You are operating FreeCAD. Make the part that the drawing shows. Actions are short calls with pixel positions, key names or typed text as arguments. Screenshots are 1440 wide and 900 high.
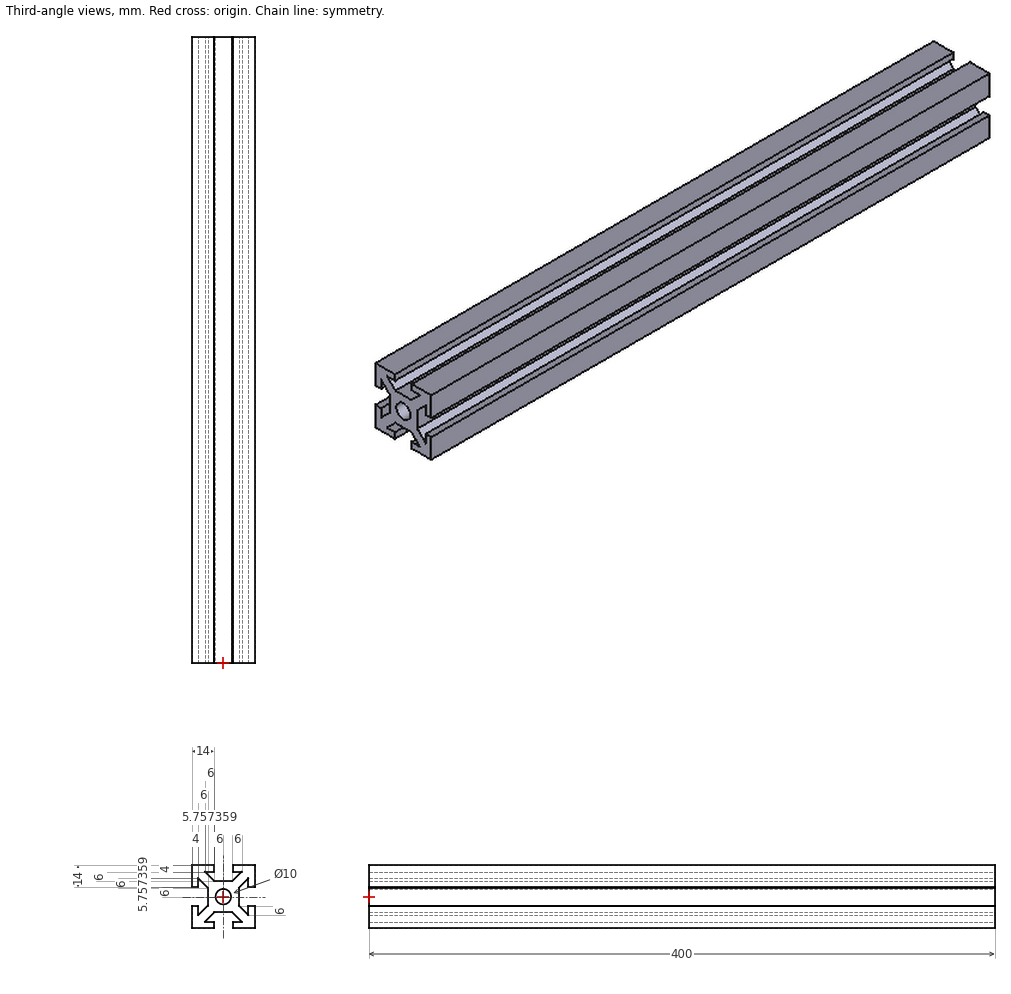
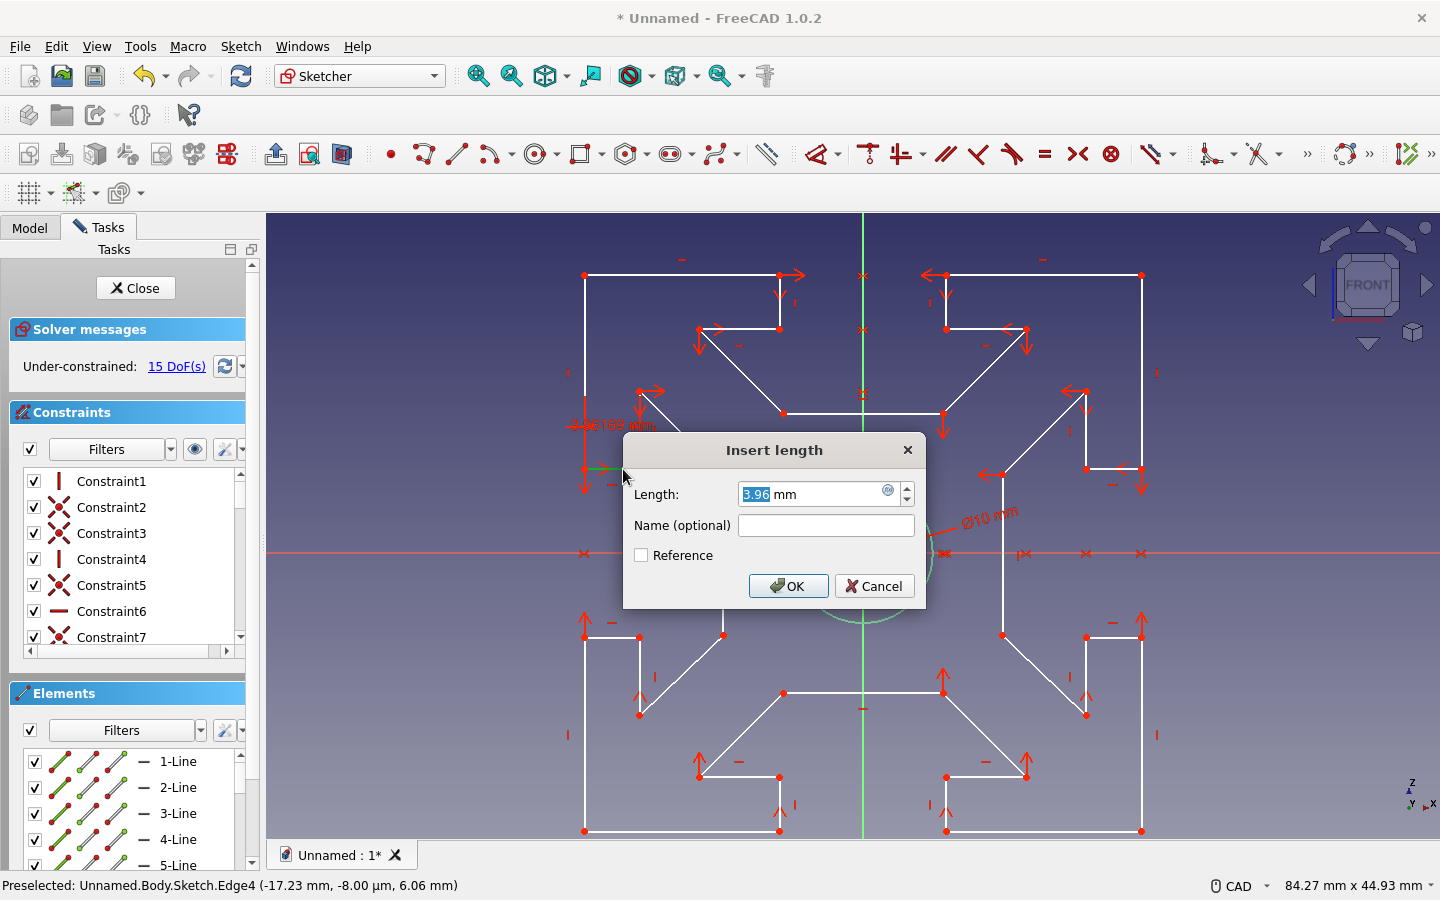
text(4)
key(Return)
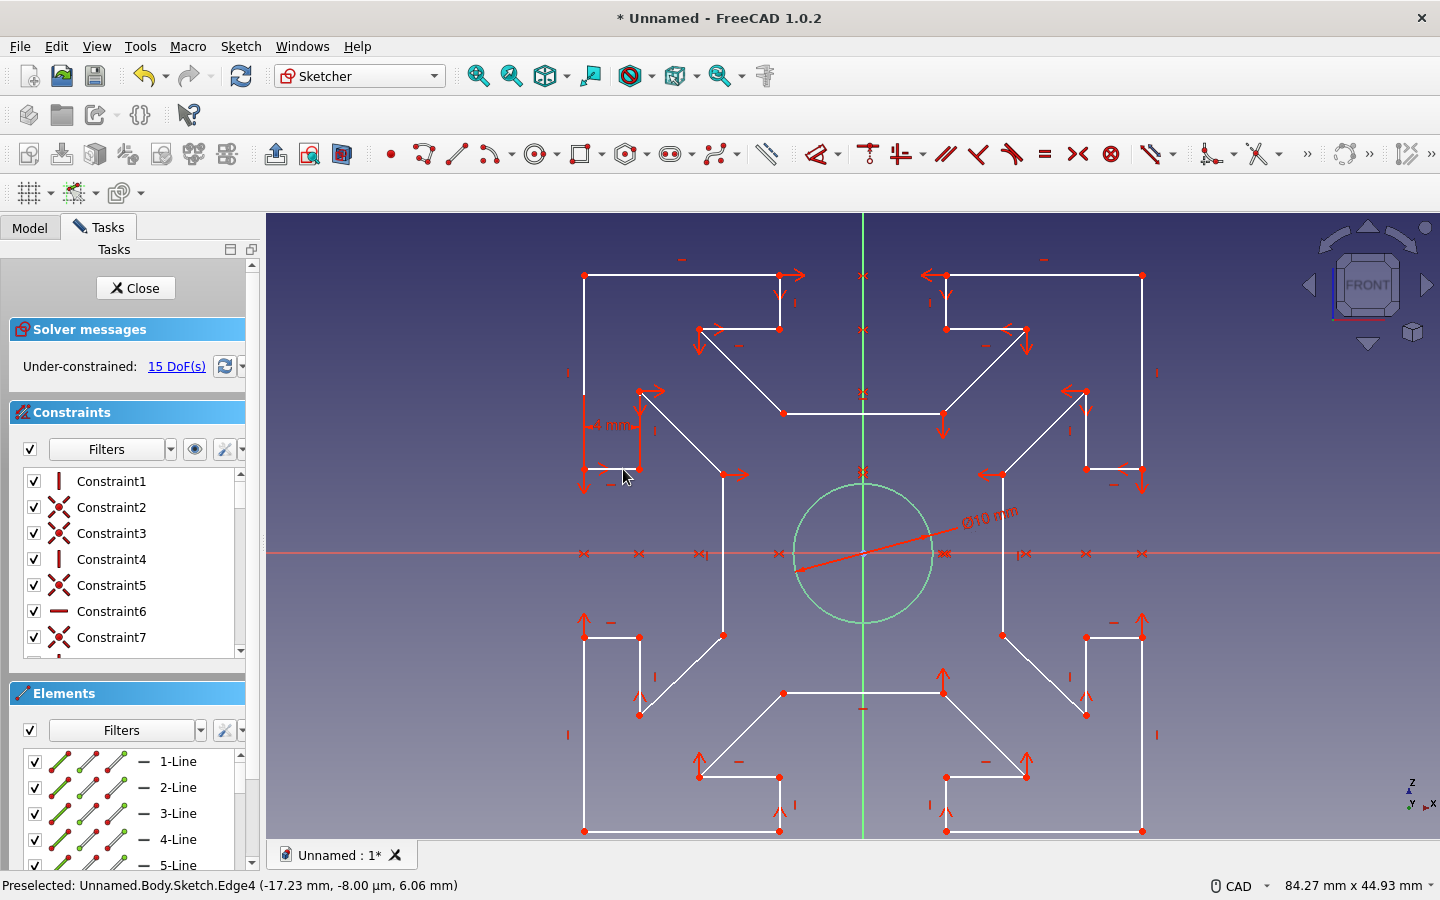
click(780, 292)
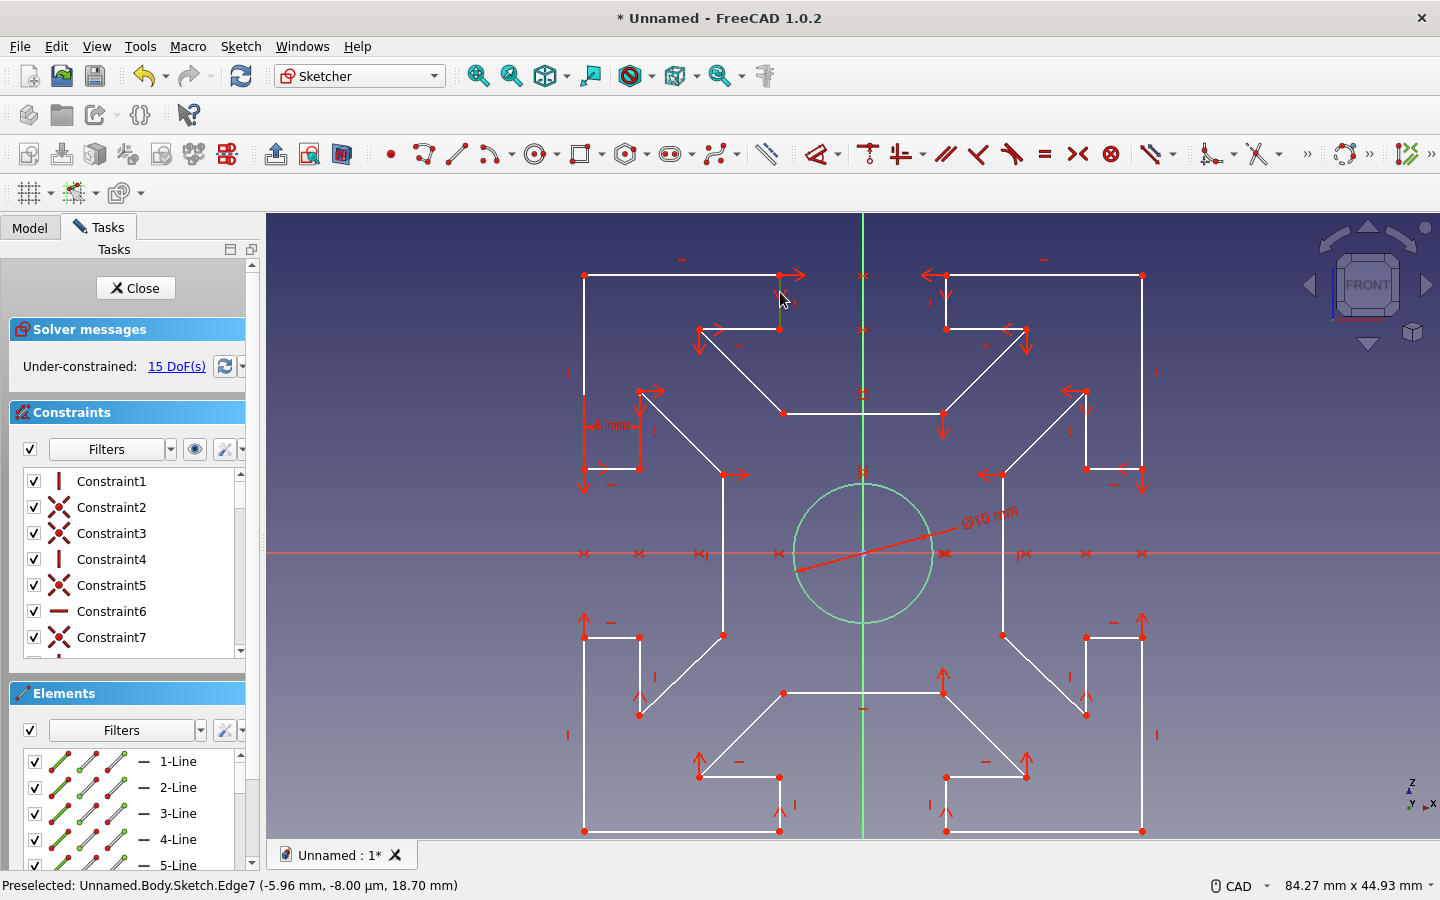
key(i)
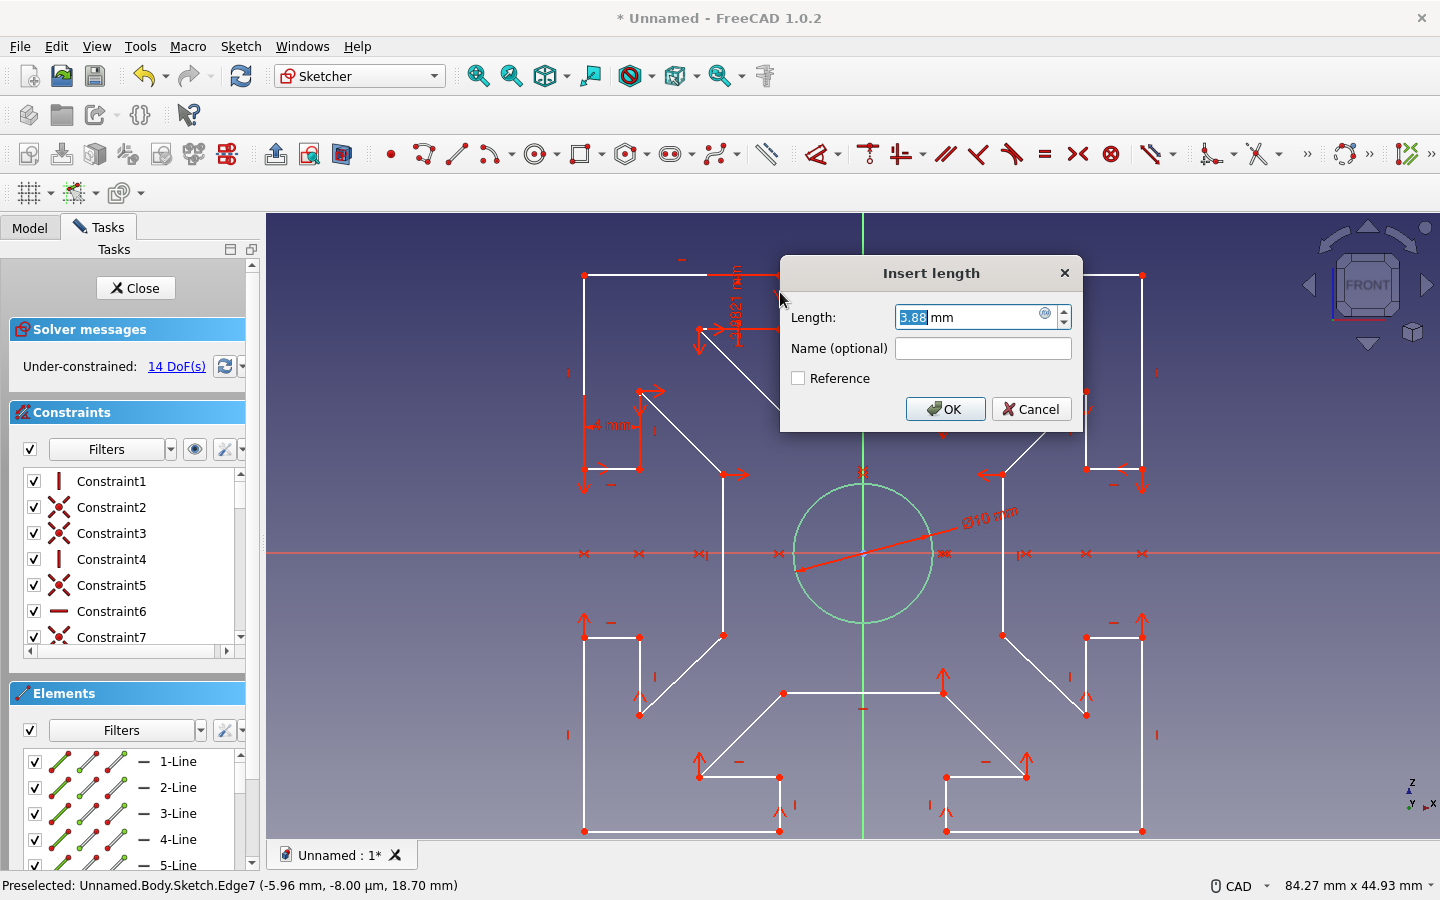
text(4)
key(Return)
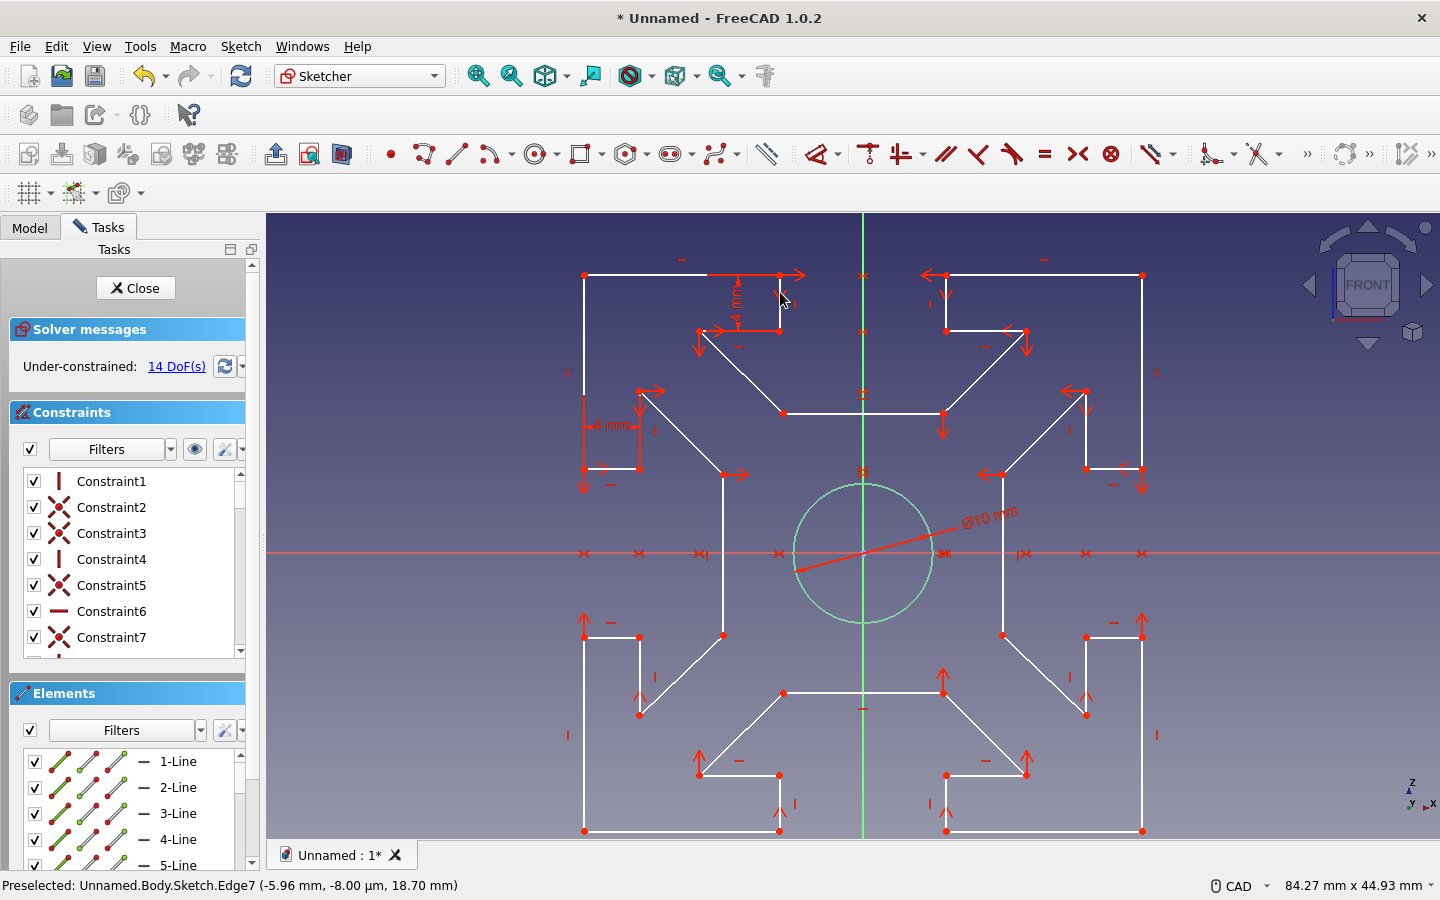
click(584, 411)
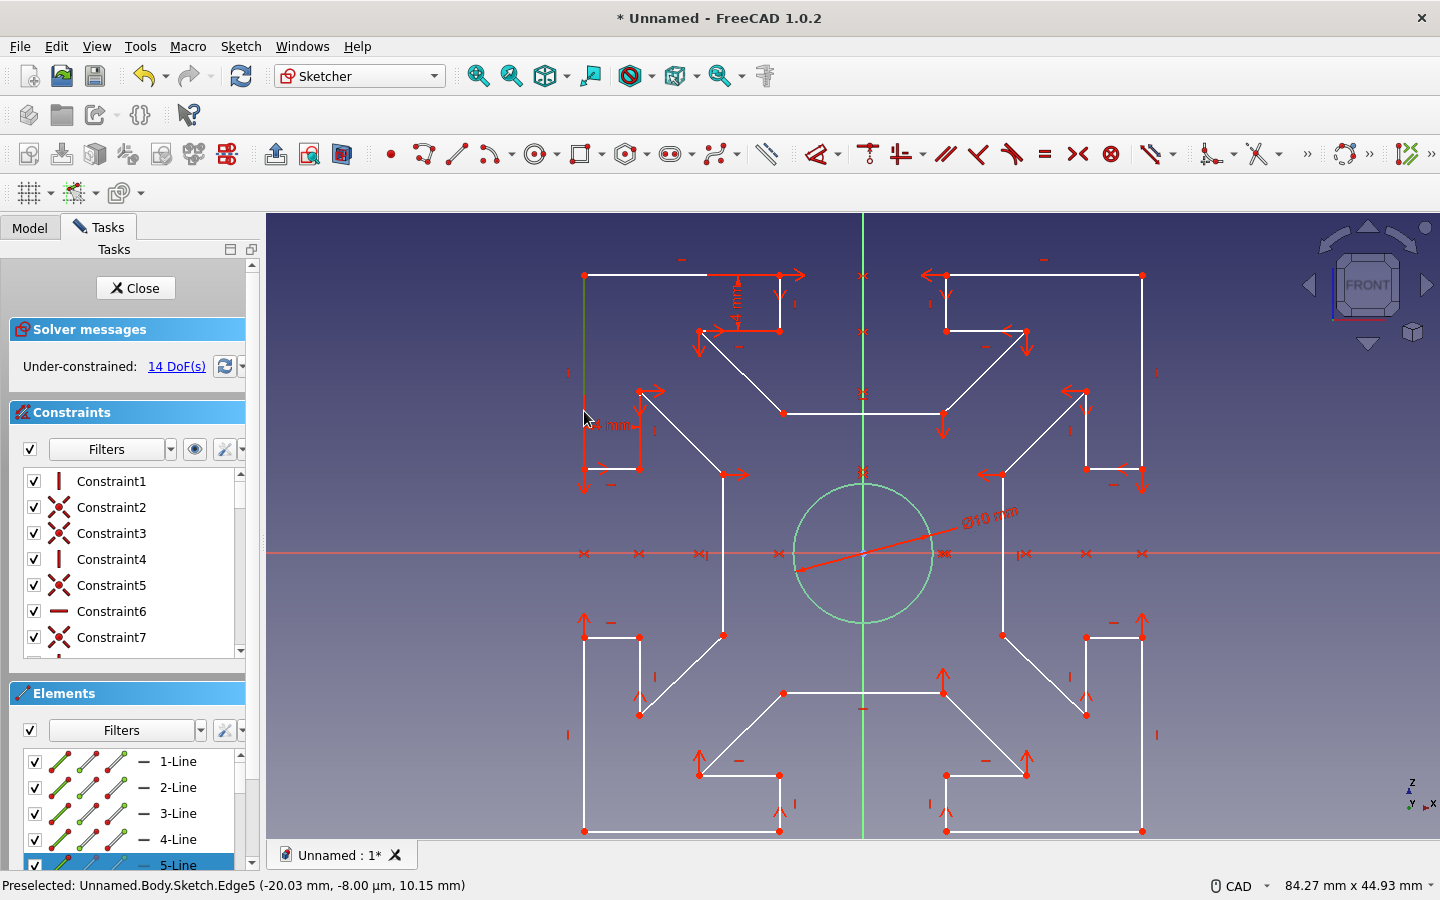
key(i)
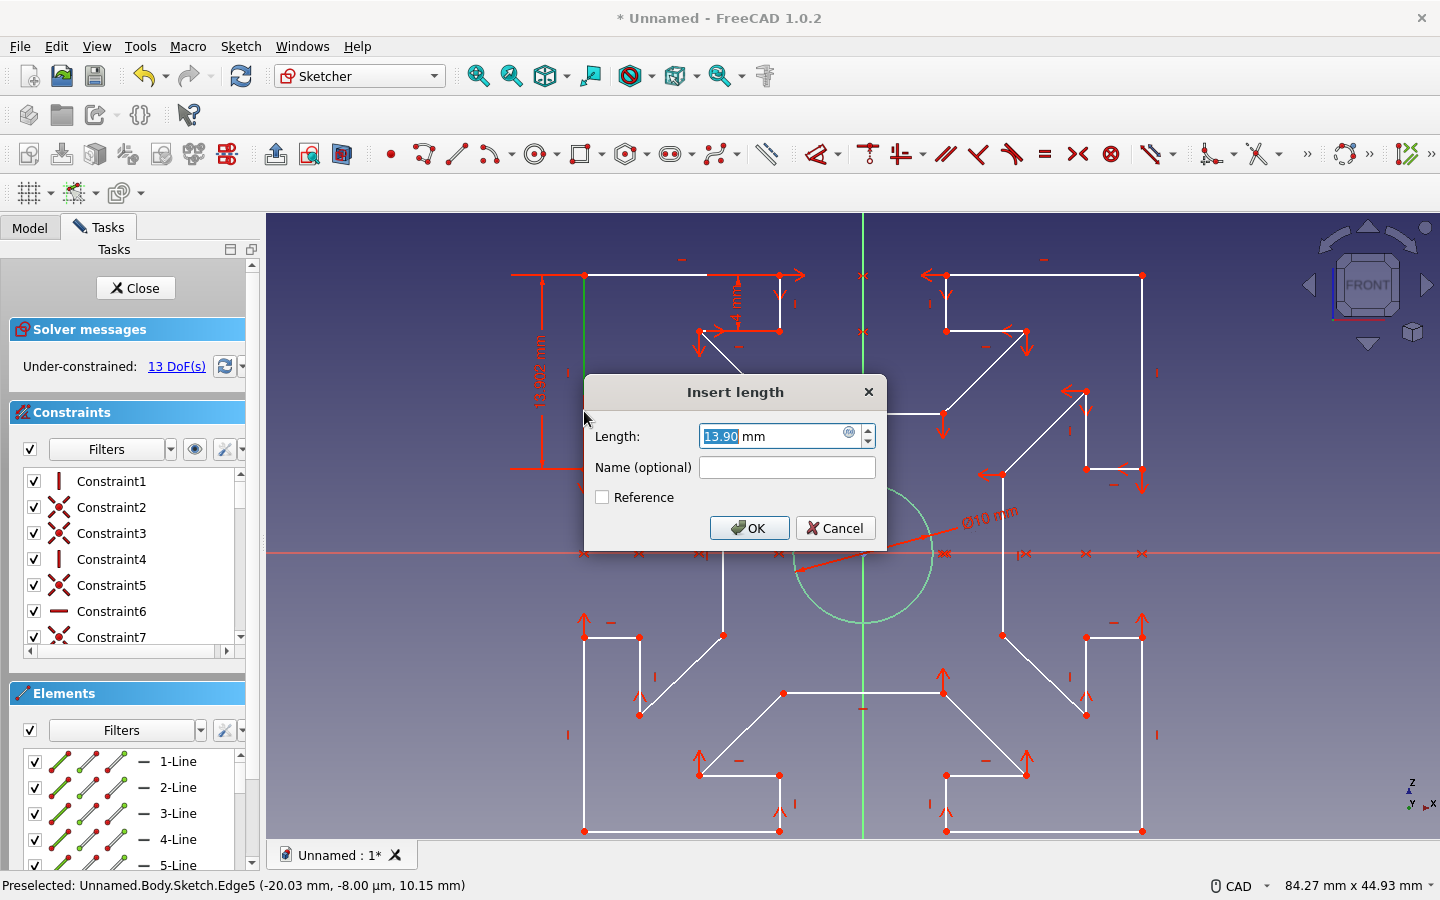
text(14)
key(Return)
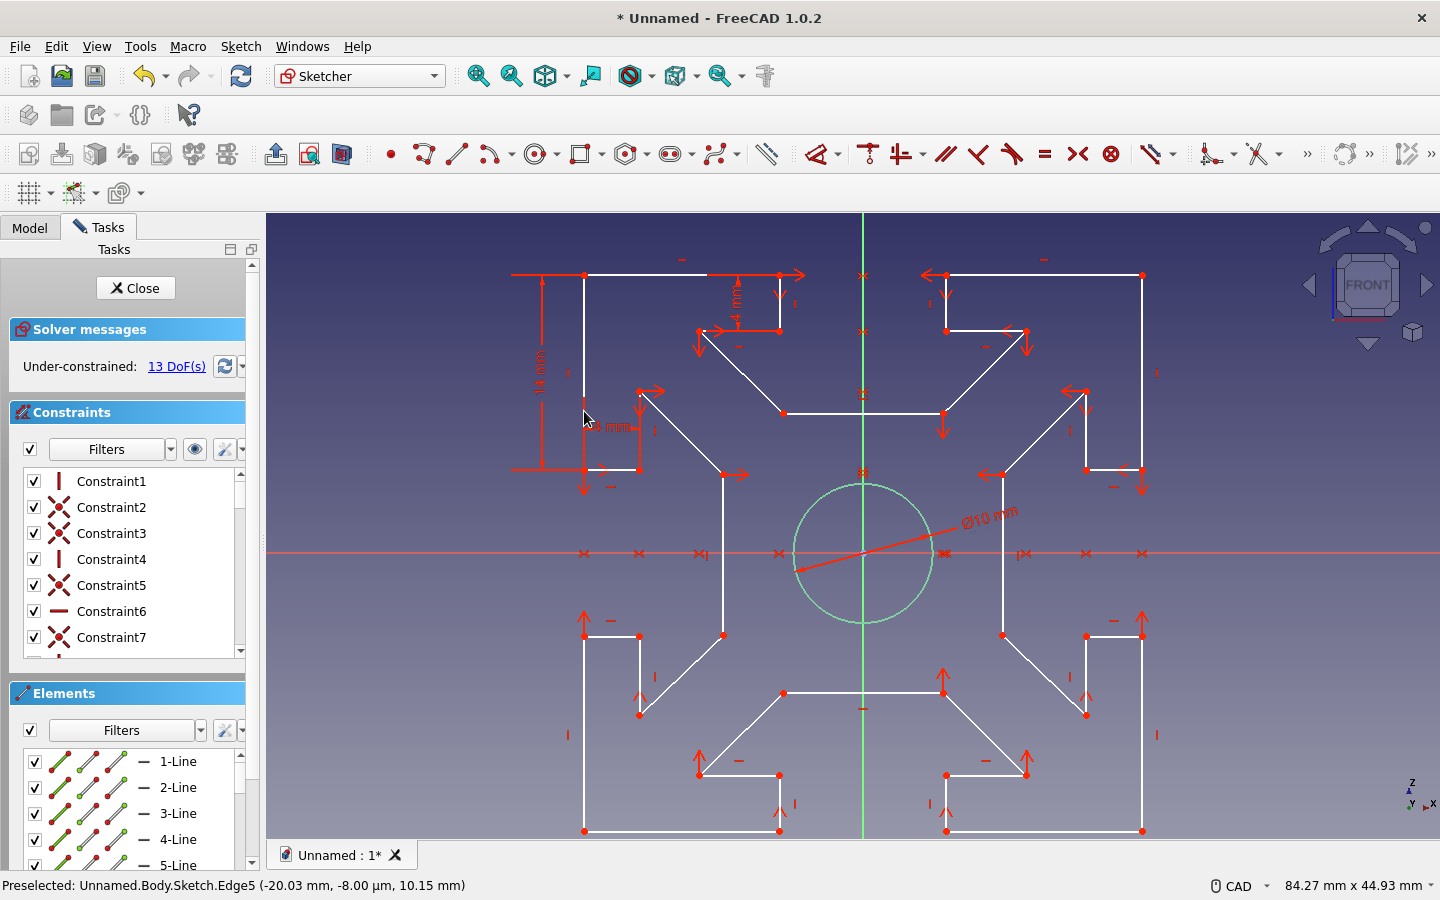
click(643, 275)